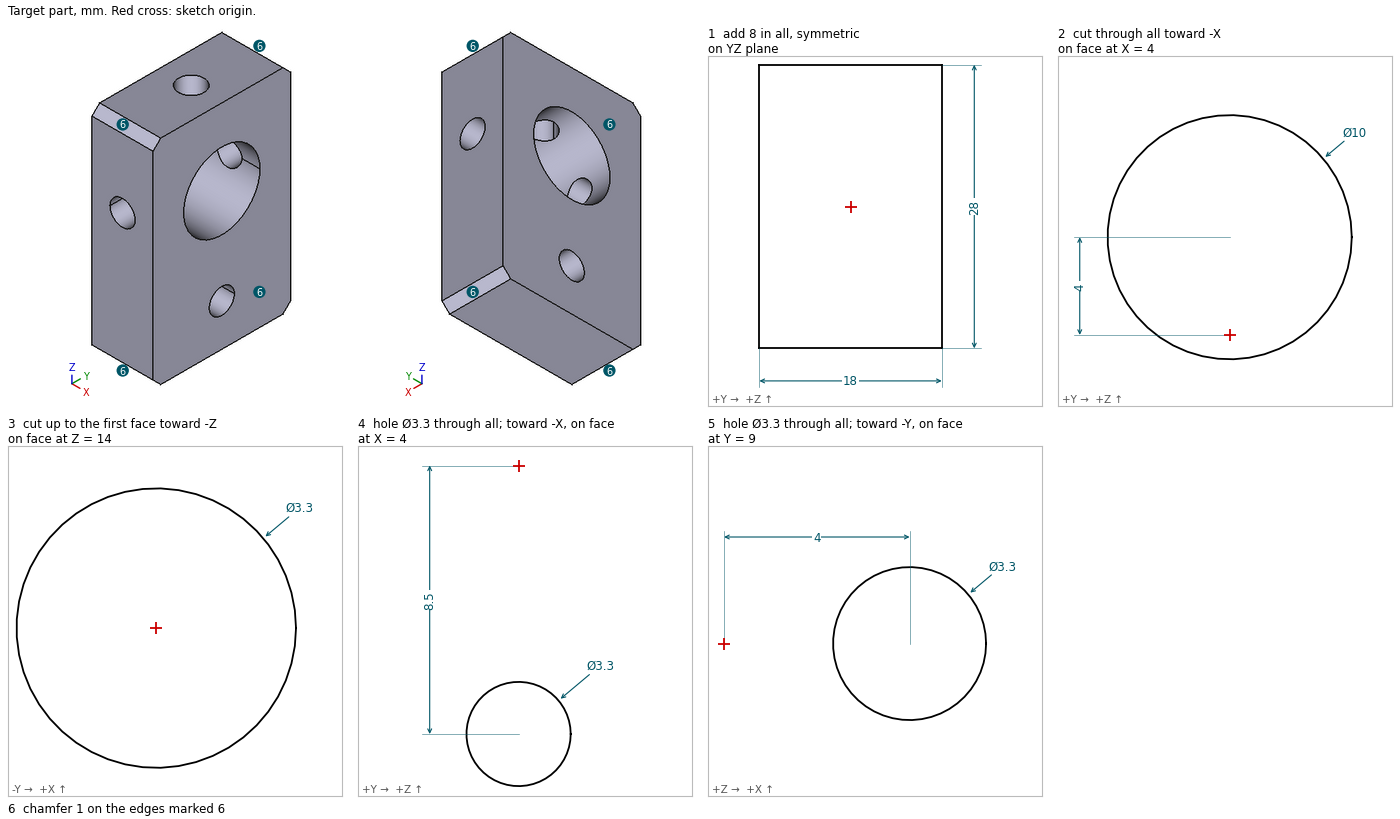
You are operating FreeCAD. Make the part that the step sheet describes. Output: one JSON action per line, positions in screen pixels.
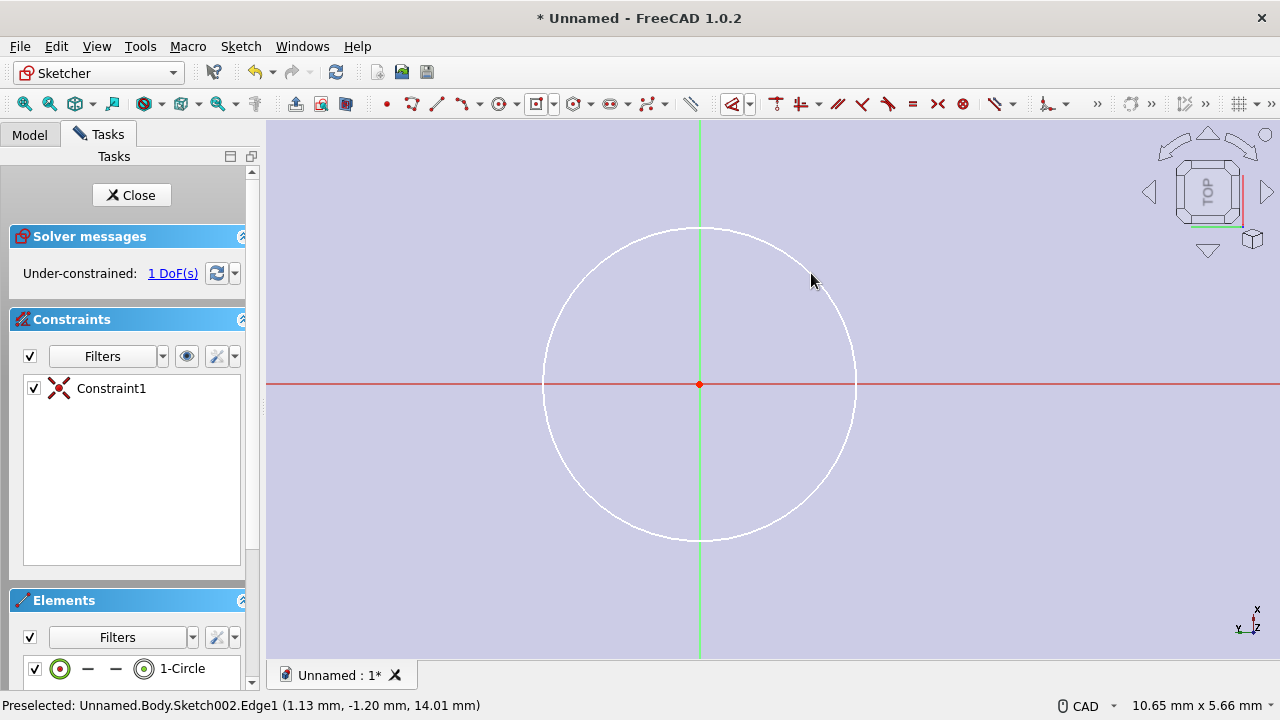
{"action": "left_click", "coordinate": [810, 273]}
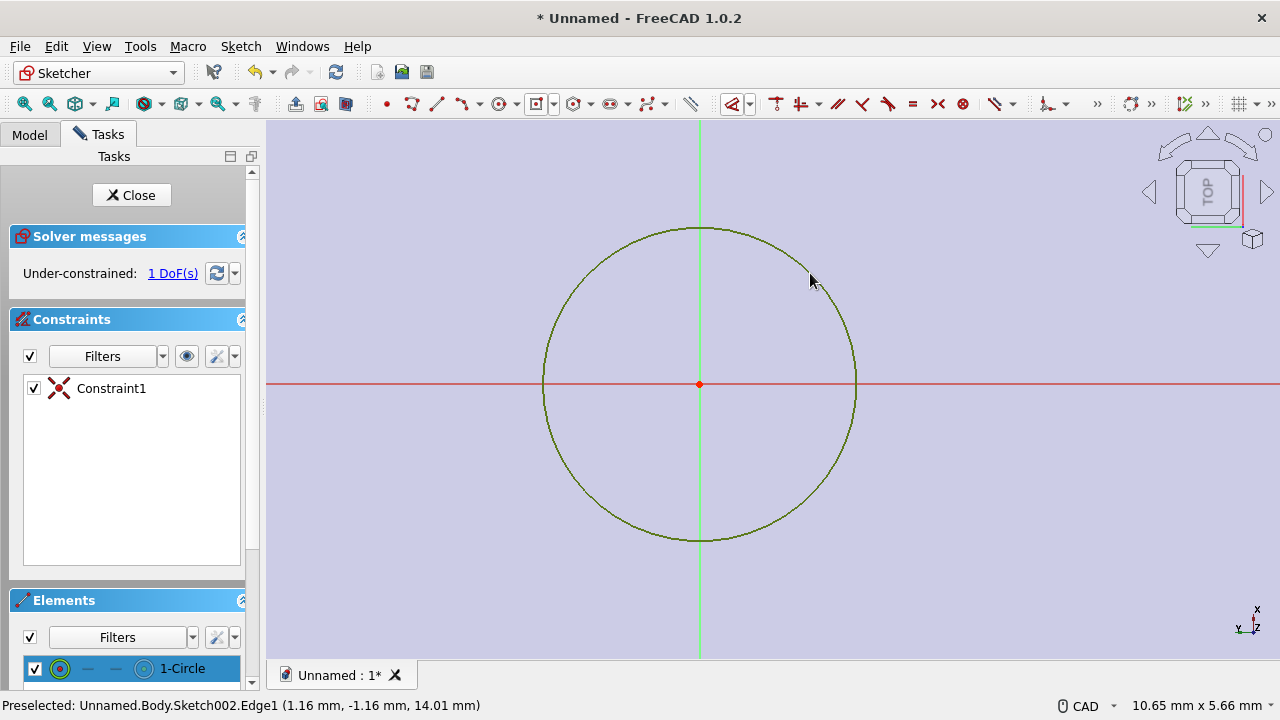
{"action": "key", "text": "k o"}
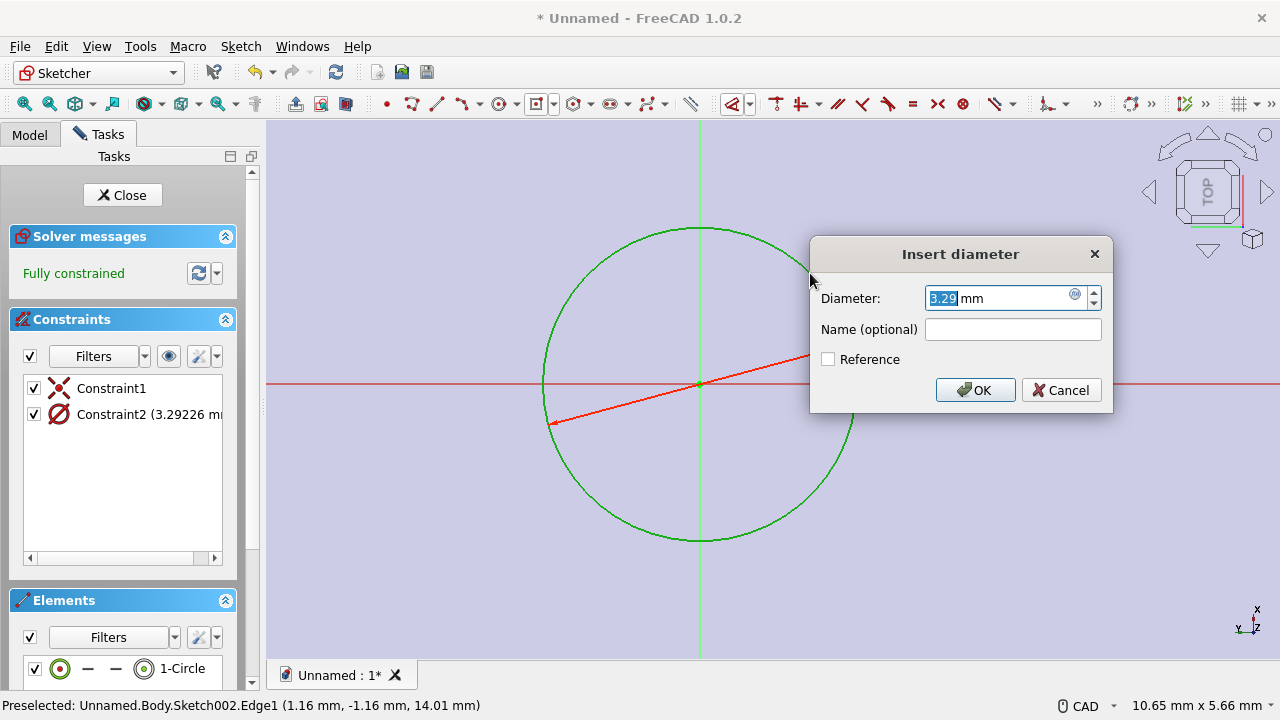
{"action": "type", "text": "3.3"}
{"action": "key", "text": "Return"}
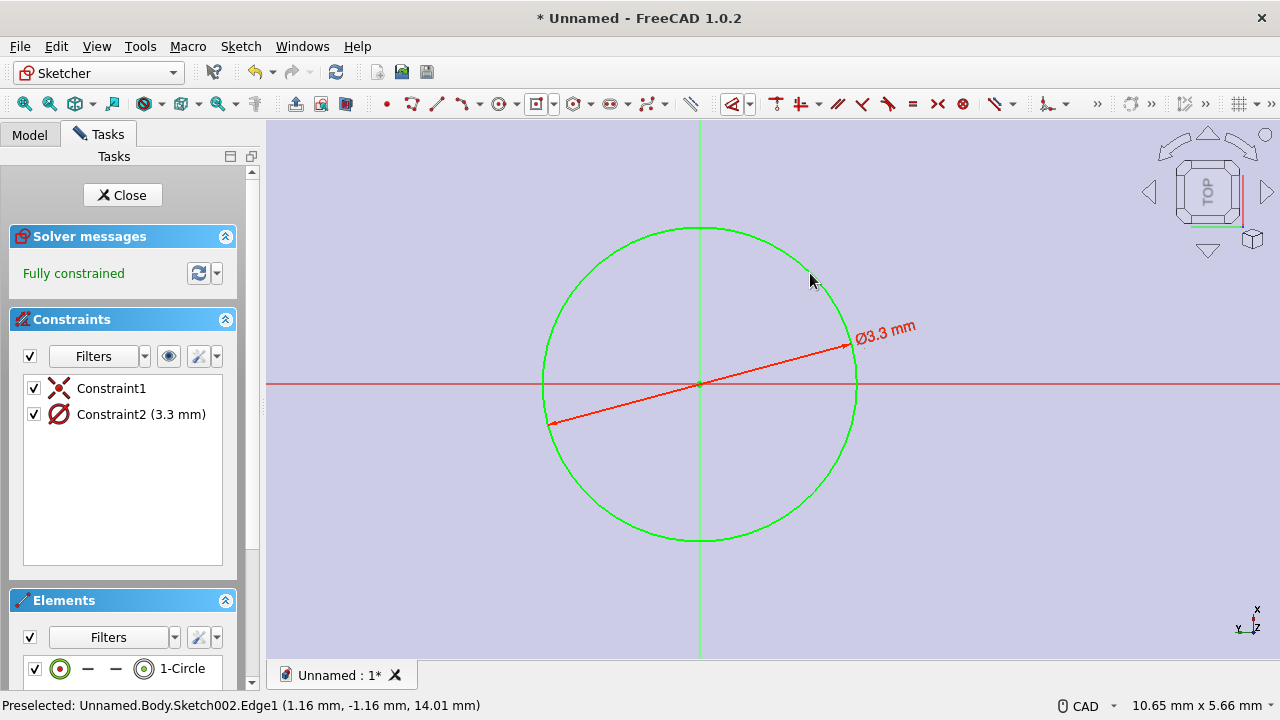
{"action": "left_click", "coordinate": [123, 195]}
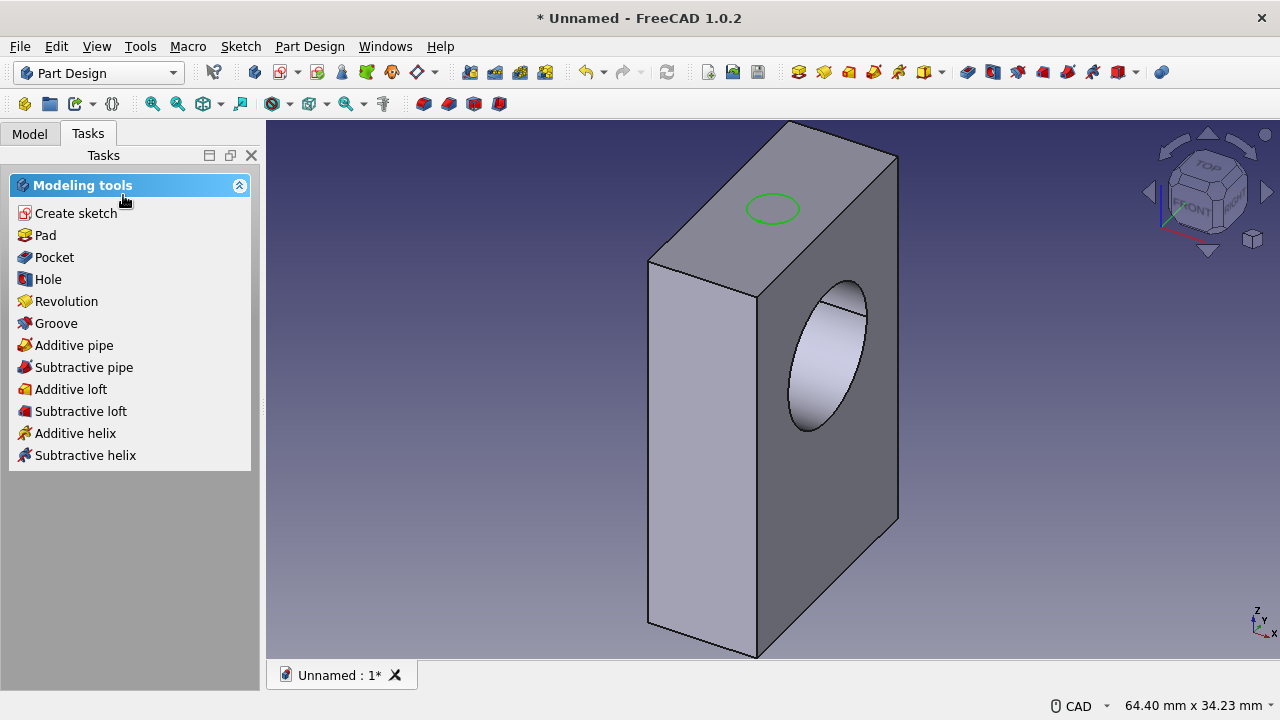
{"action": "left_click", "coordinate": [968, 72]}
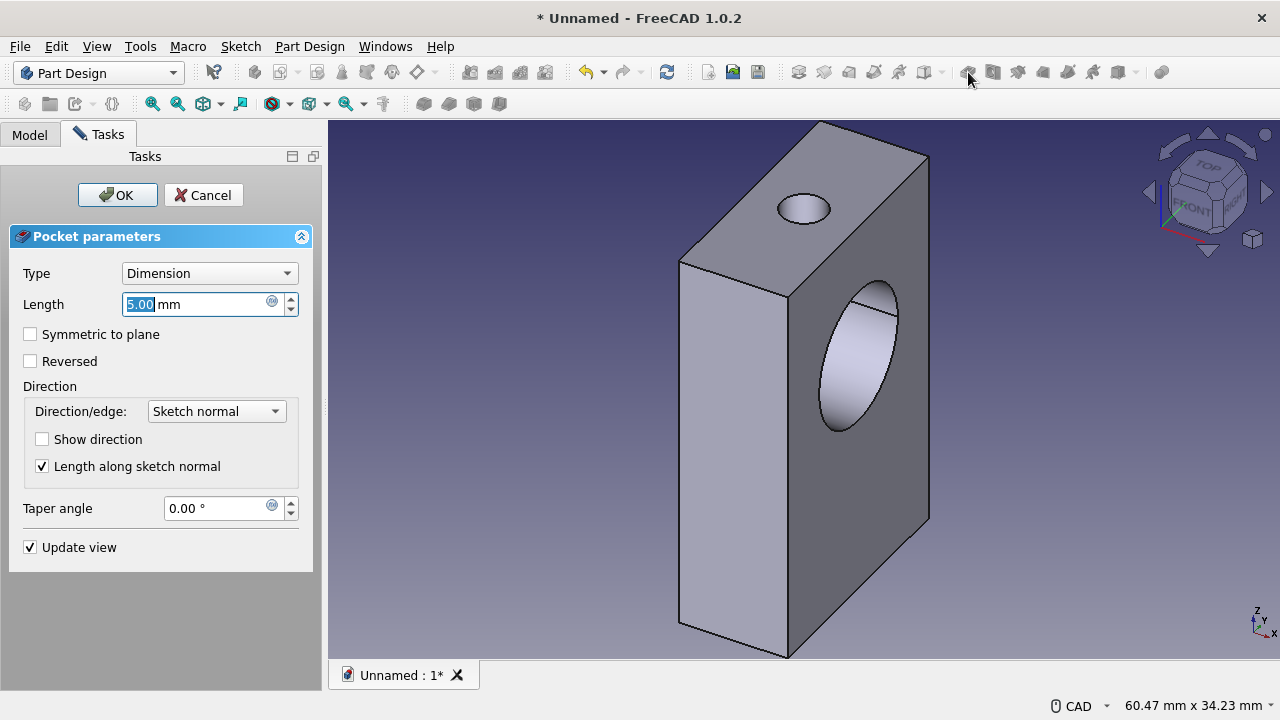
{"action": "left_click", "coordinate": [210, 274]}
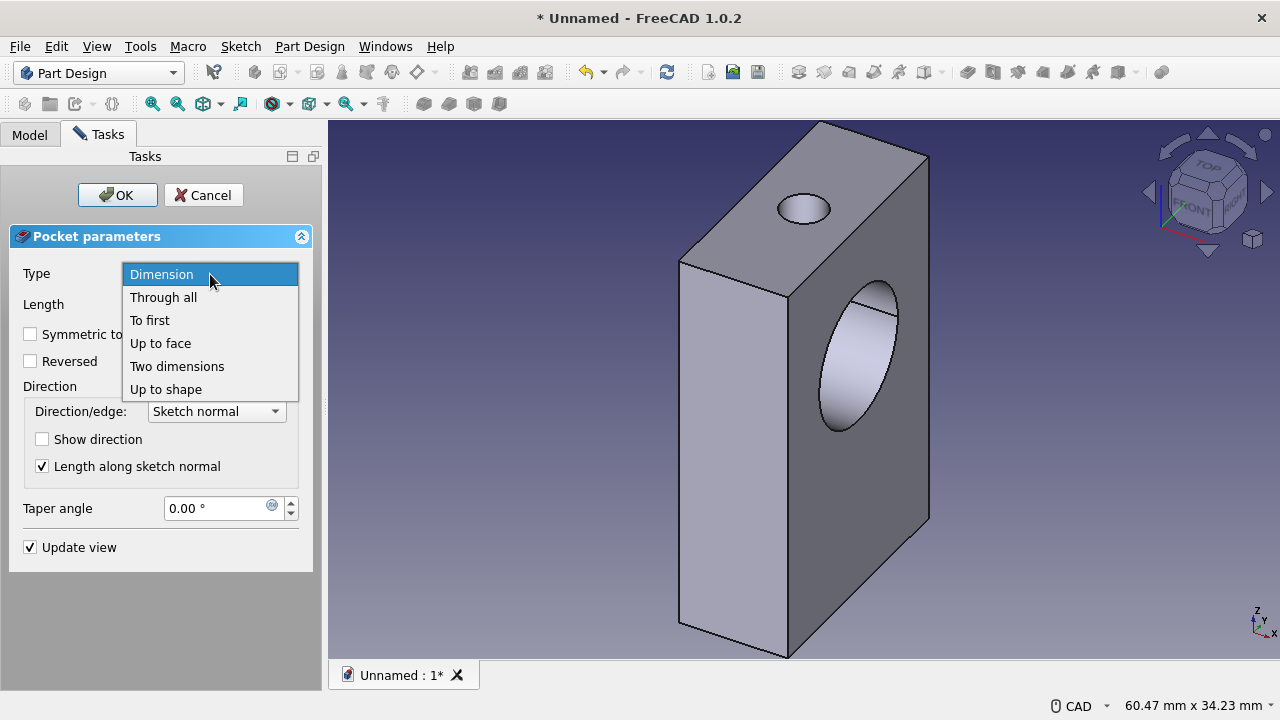
{"action": "left_click", "coordinate": [208, 320]}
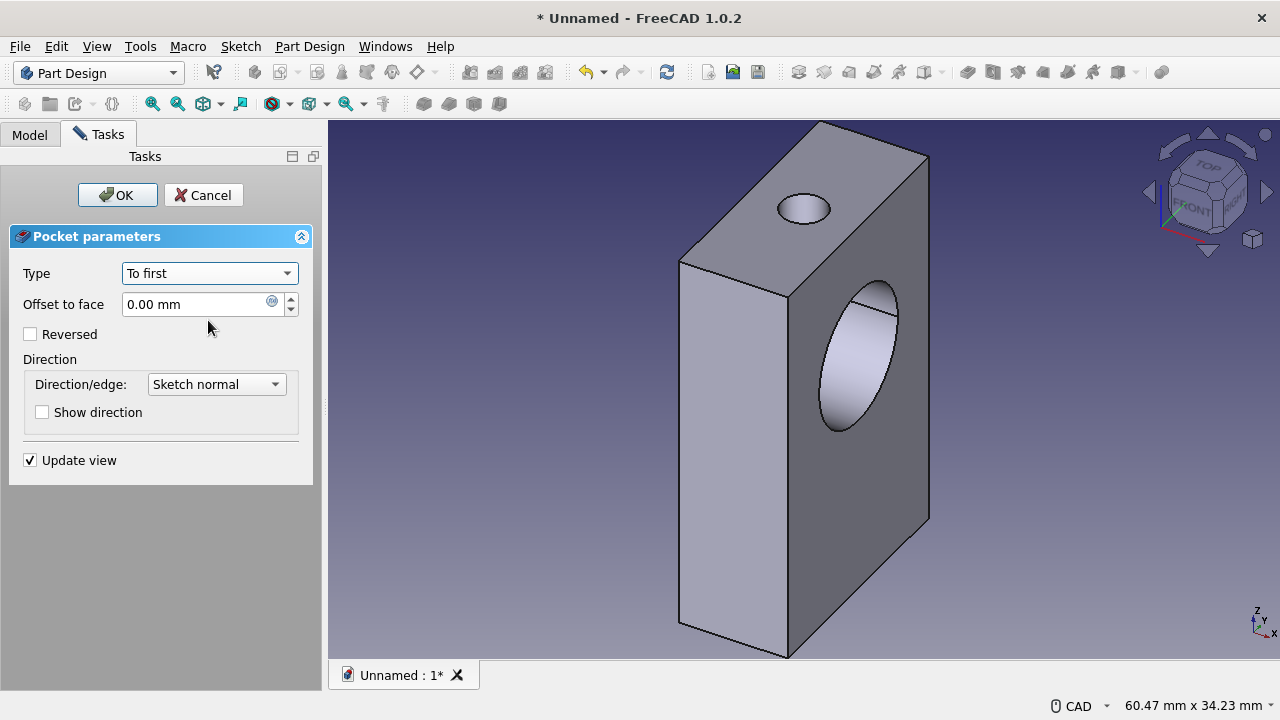
{"action": "left_click", "coordinate": [118, 195]}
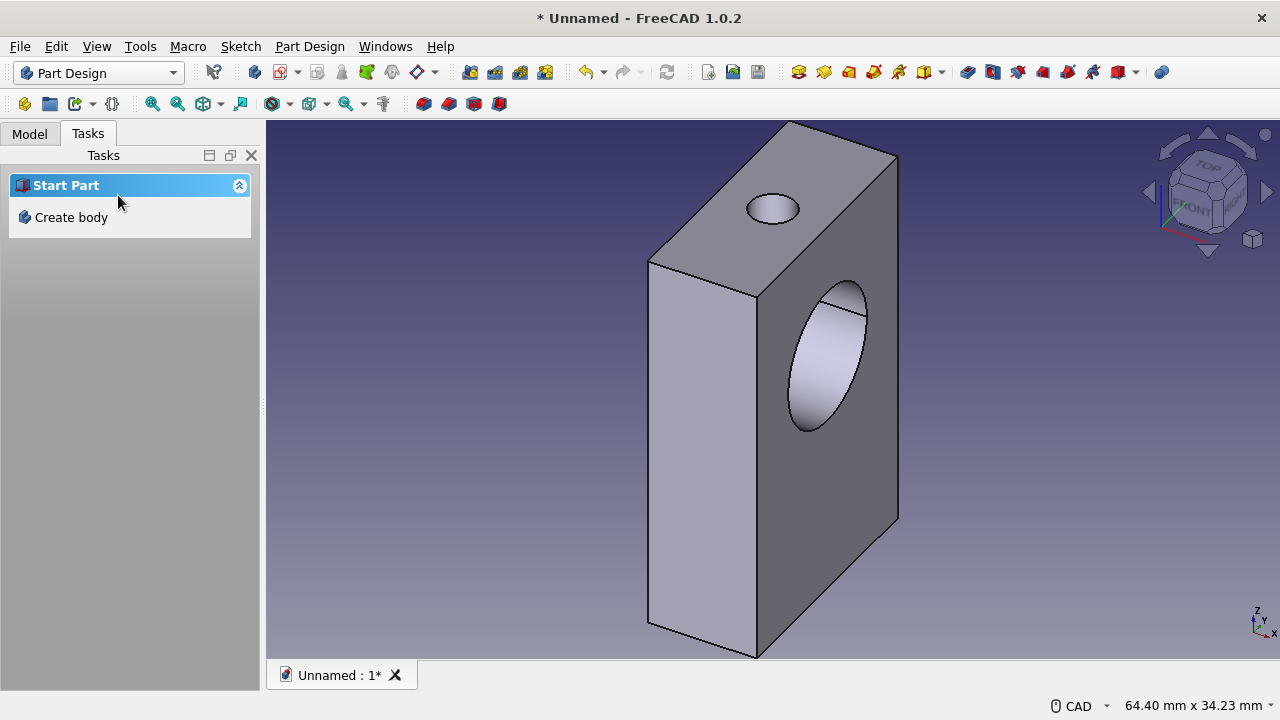
{"action": "left_click", "coordinate": [153, 104]}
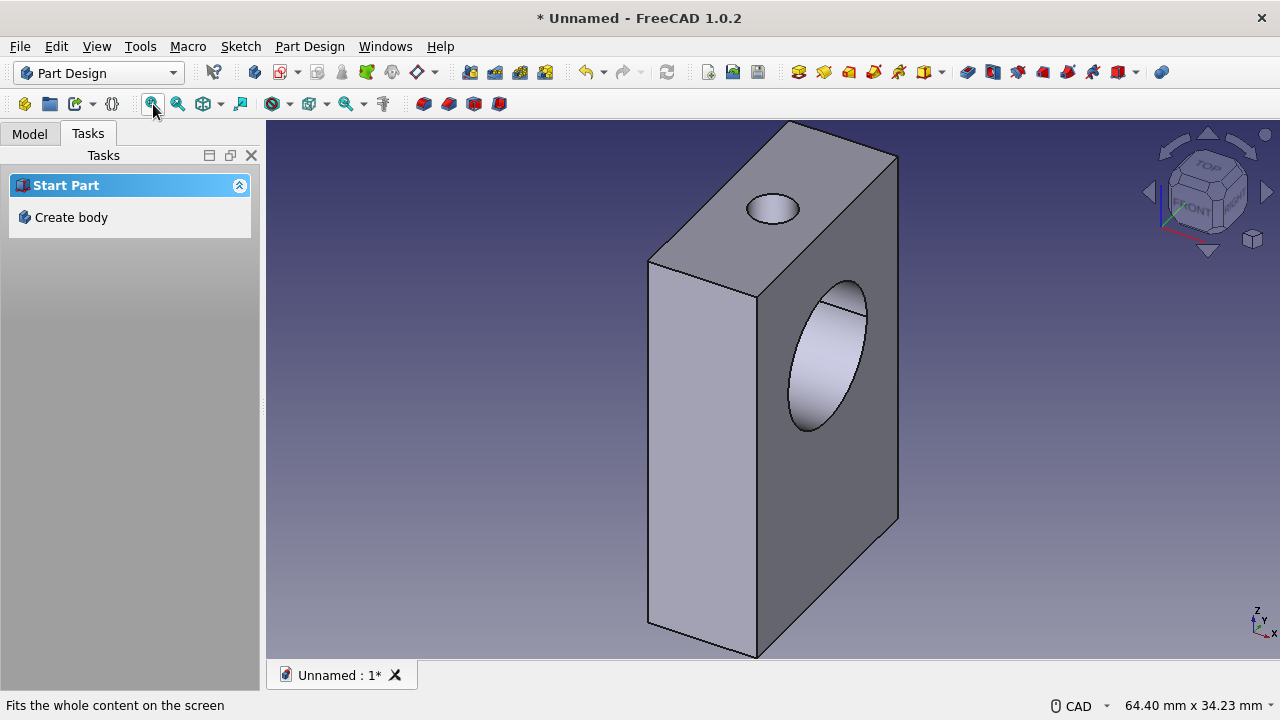
{"action": "left_click", "coordinate": [848, 490]}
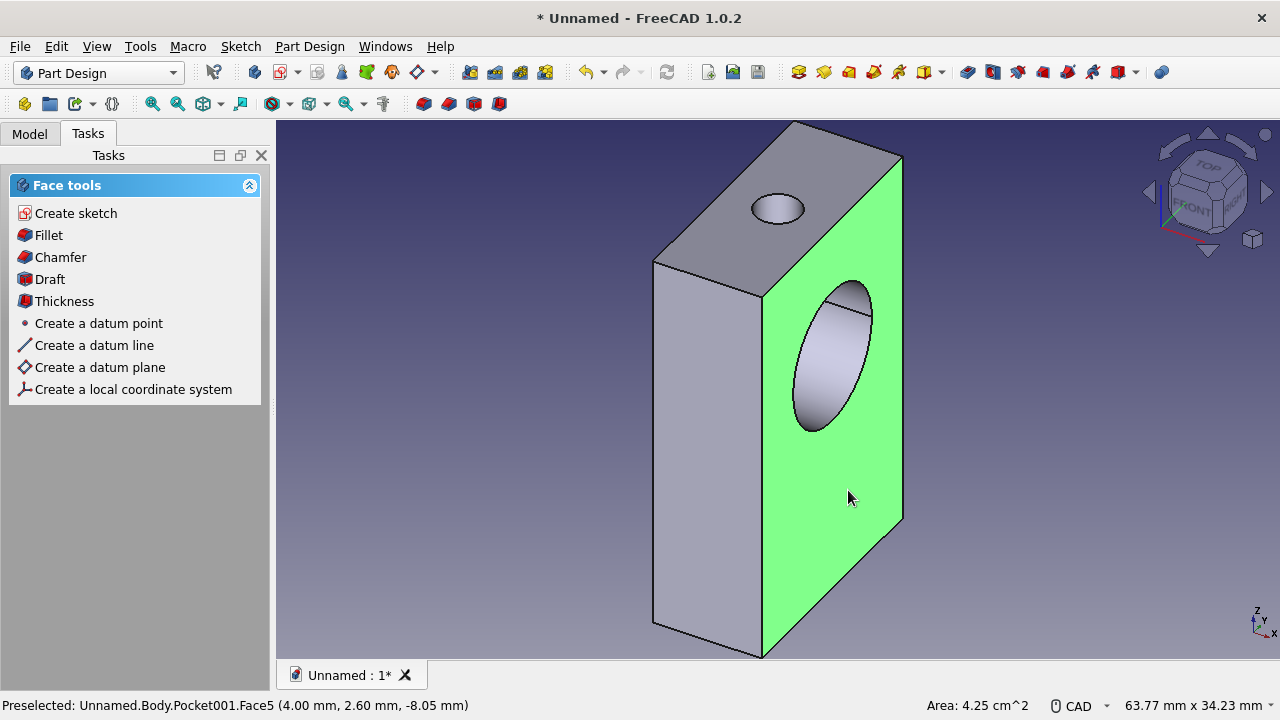
{"action": "left_click", "coordinate": [280, 72]}